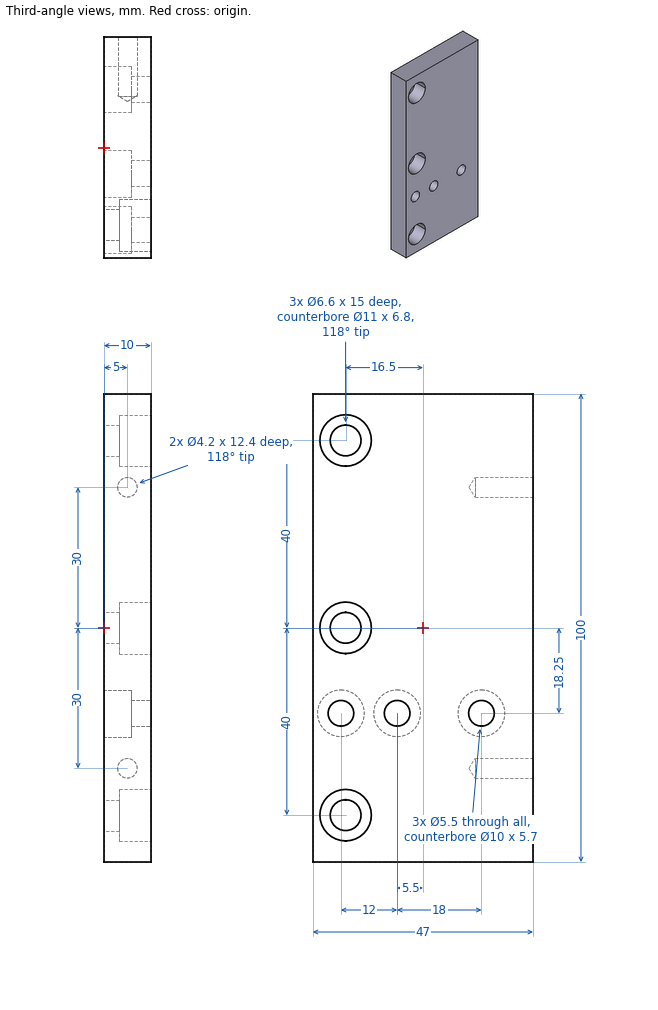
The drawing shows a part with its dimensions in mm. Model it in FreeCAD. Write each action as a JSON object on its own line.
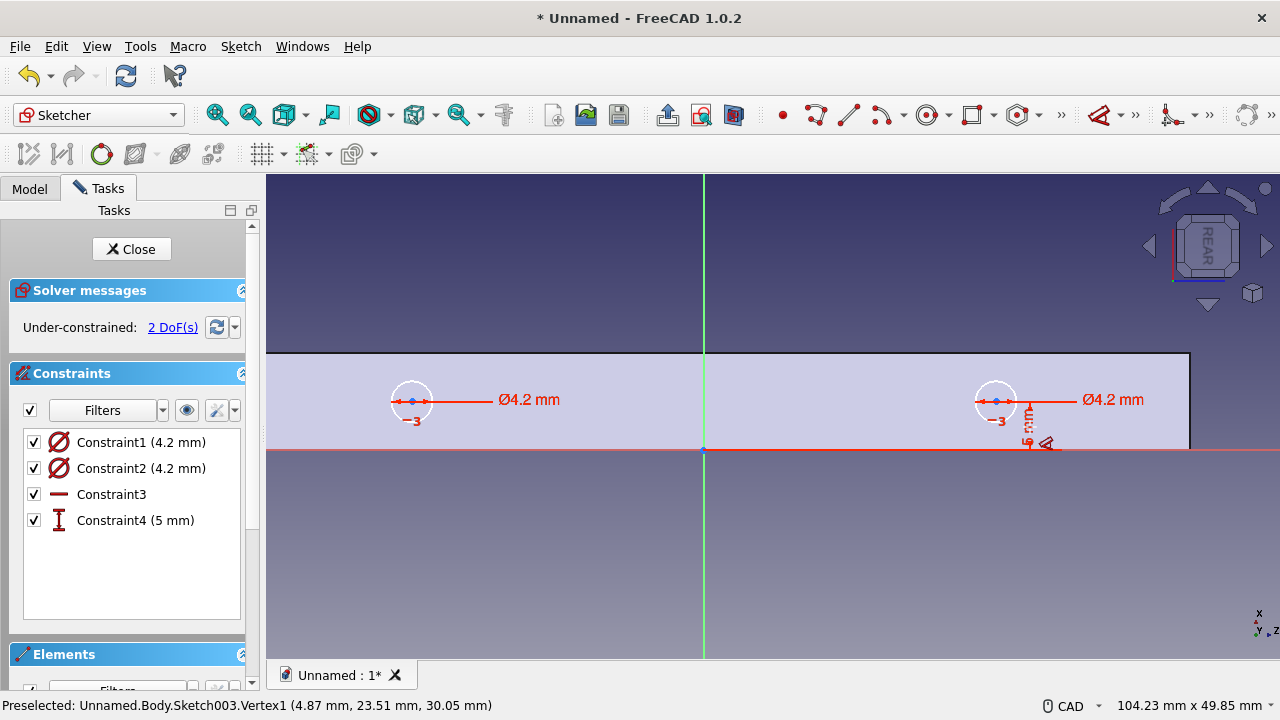
{"action": "left_click", "coordinate": [996, 402]}
{"action": "left_click", "coordinate": [850, 484]}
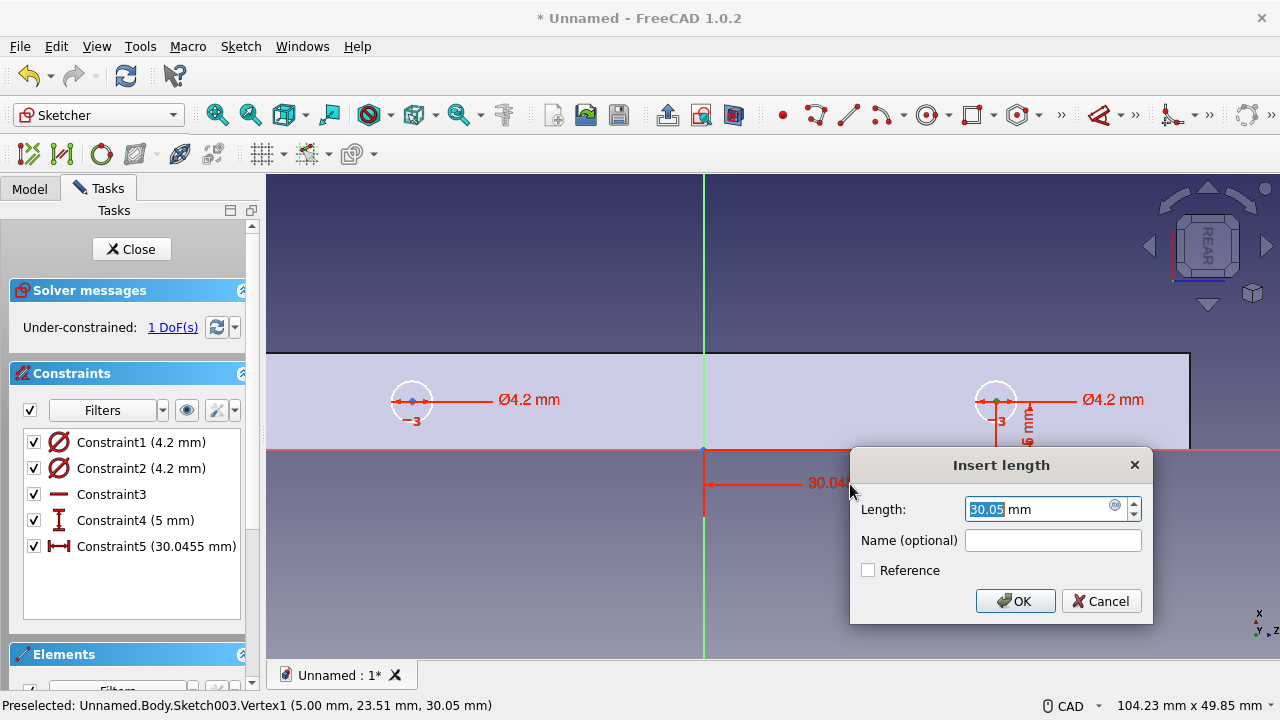
{"action": "type", "text": "30"}
{"action": "key", "text": "Return"}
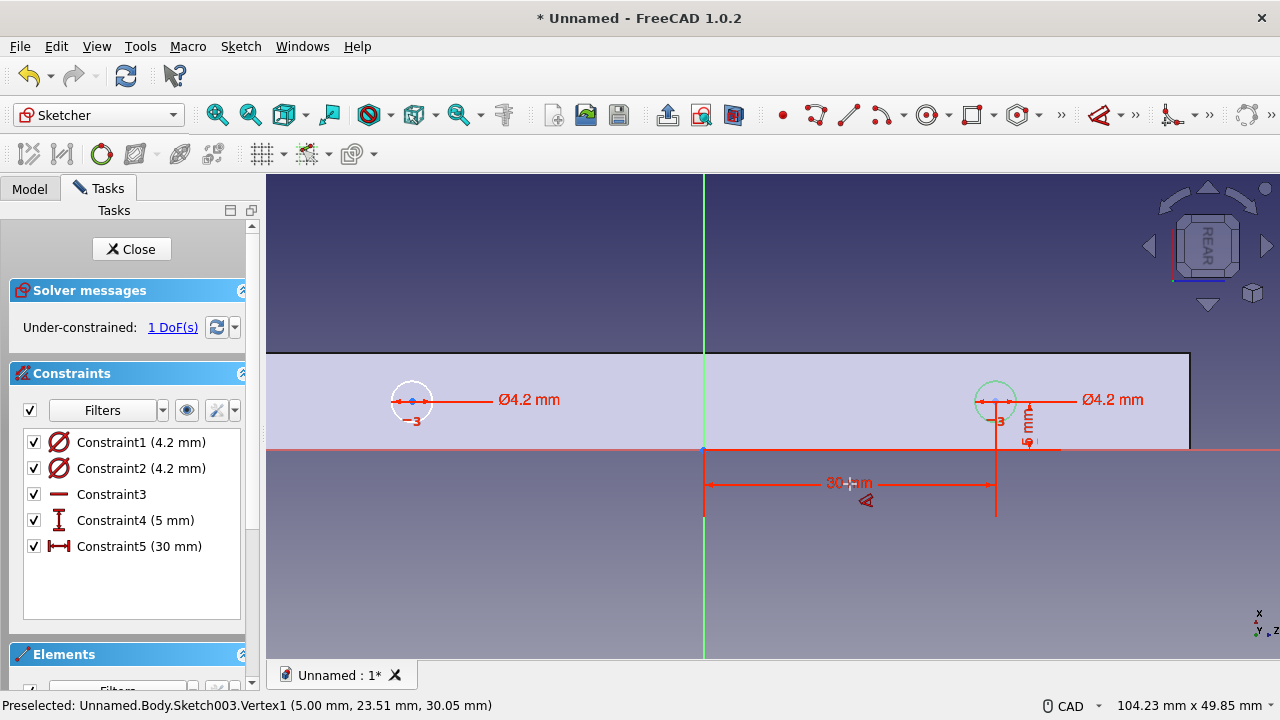
{"action": "left_click", "coordinate": [412, 402]}
{"action": "left_click", "coordinate": [558, 484]}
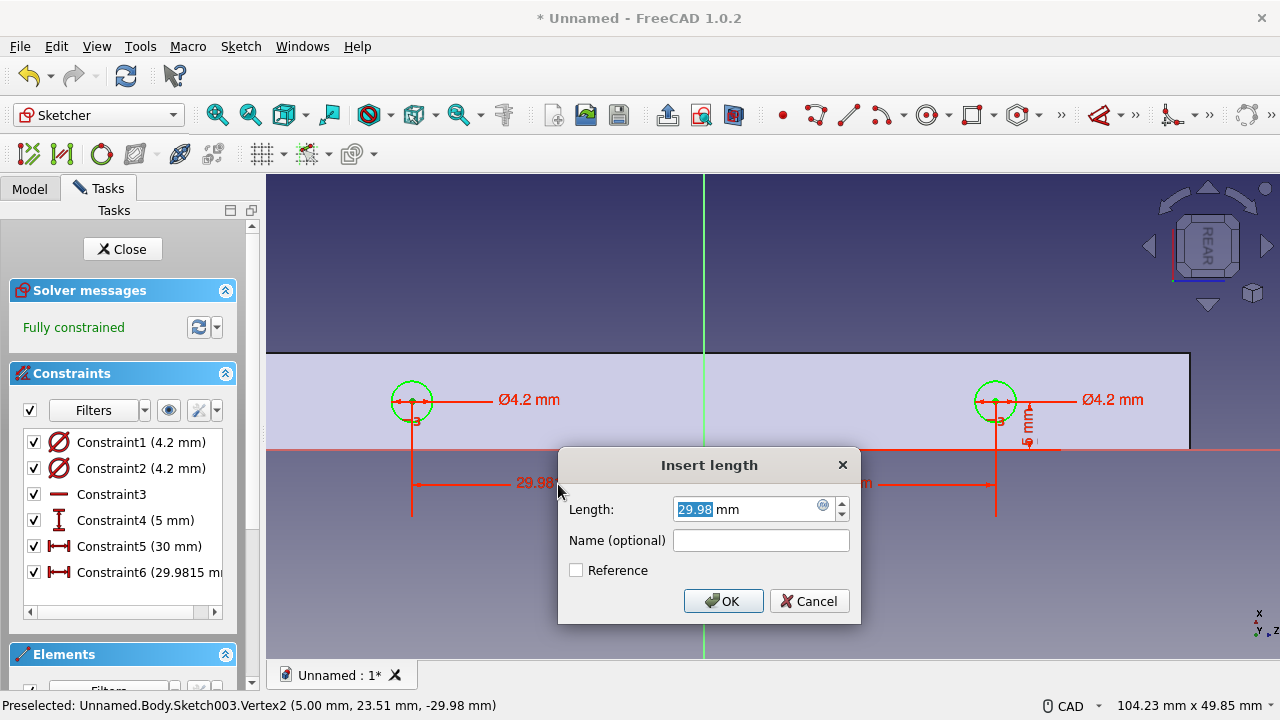
{"action": "type", "text": "30"}
{"action": "key", "text": "Return"}
{"action": "key", "text": "Escape"}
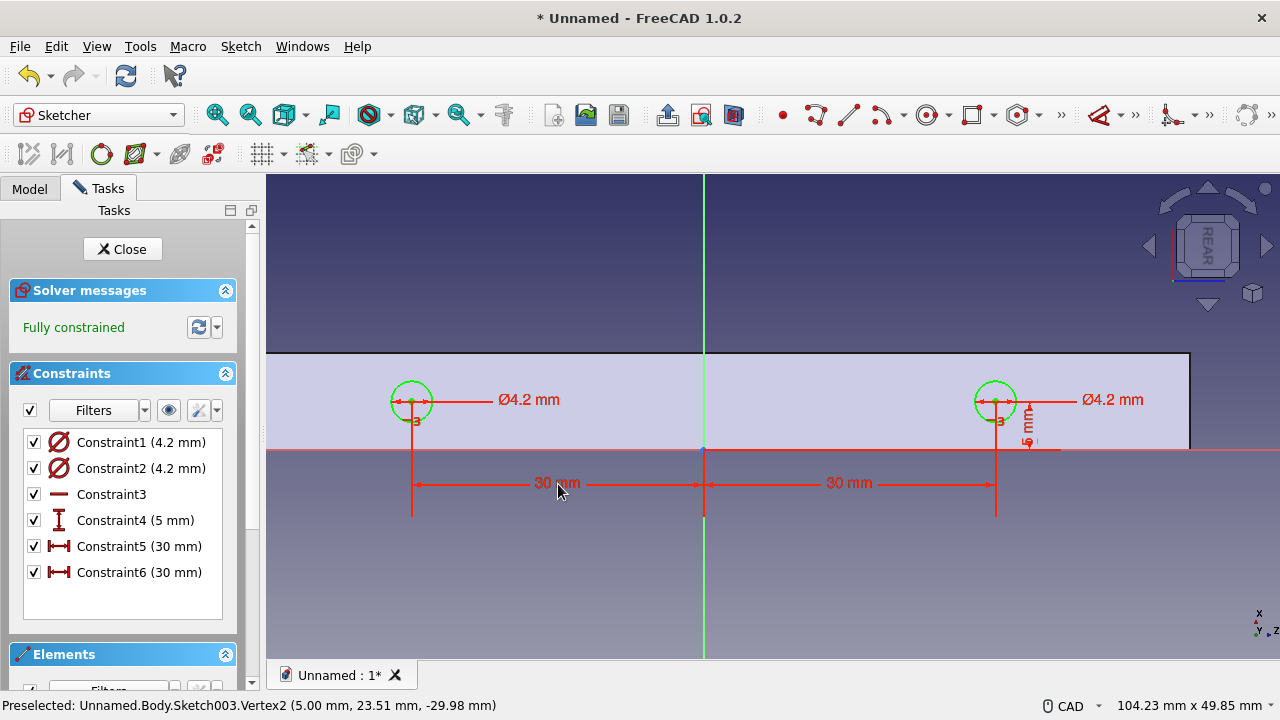
{"action": "left_click", "coordinate": [123, 249]}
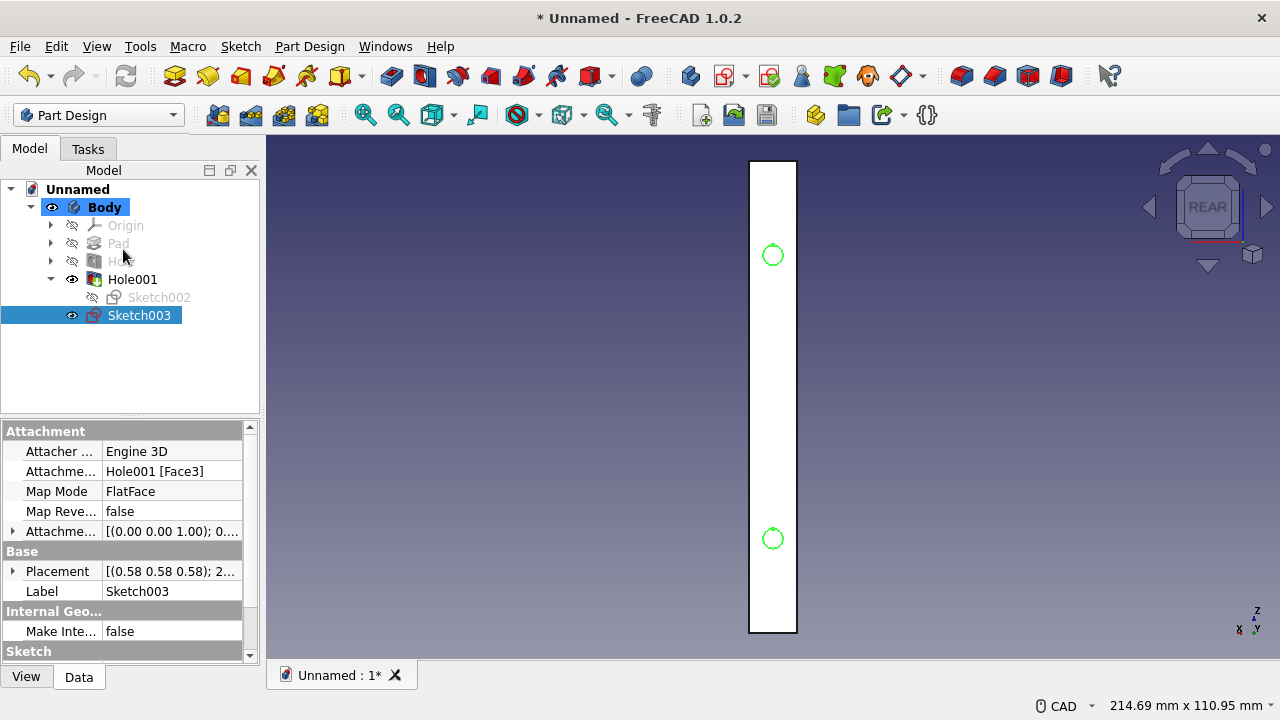
{"action": "left_click", "coordinate": [425, 76]}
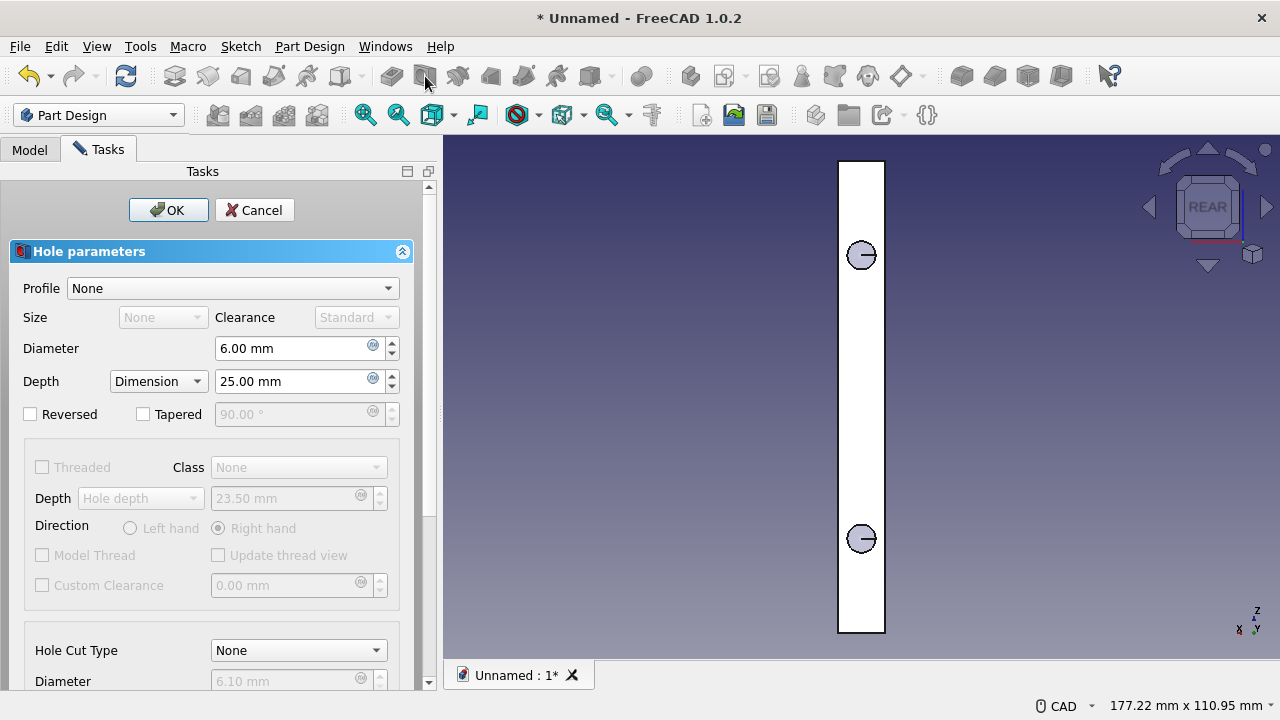
{"action": "triple_click", "coordinate": [300, 348]}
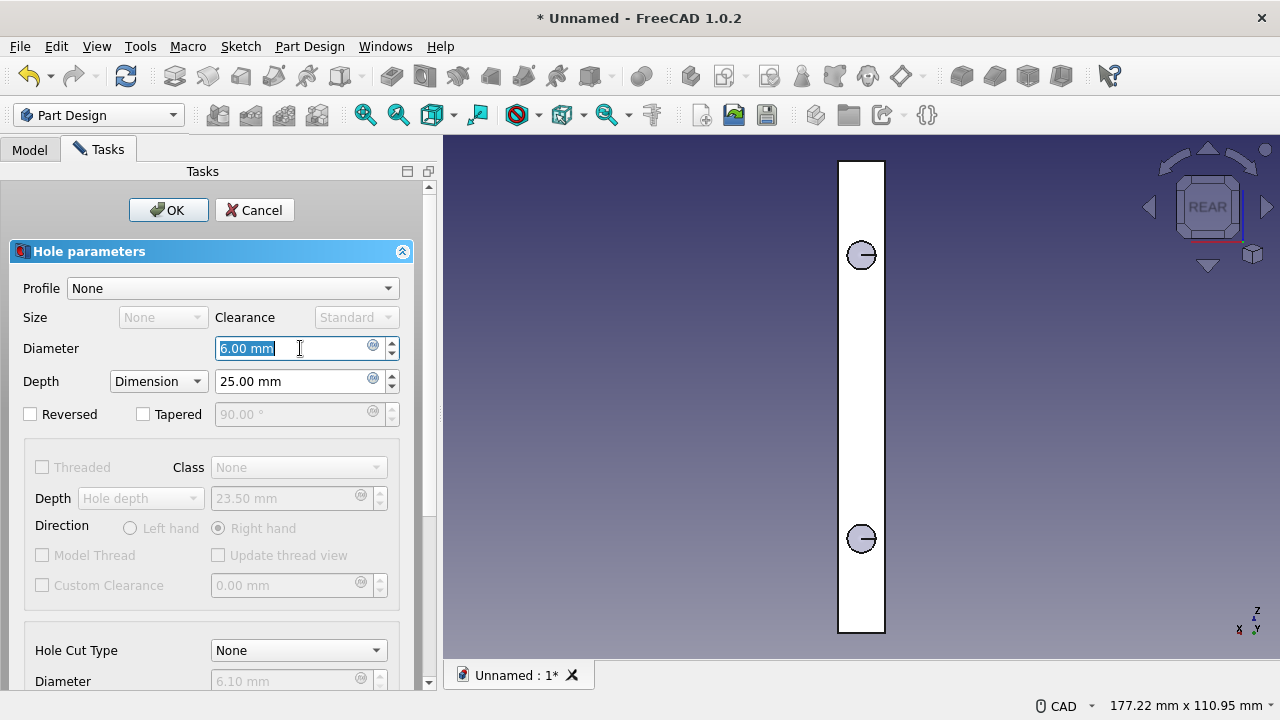
{"action": "type", "text": "4.2"}
{"action": "key", "text": "Tab"}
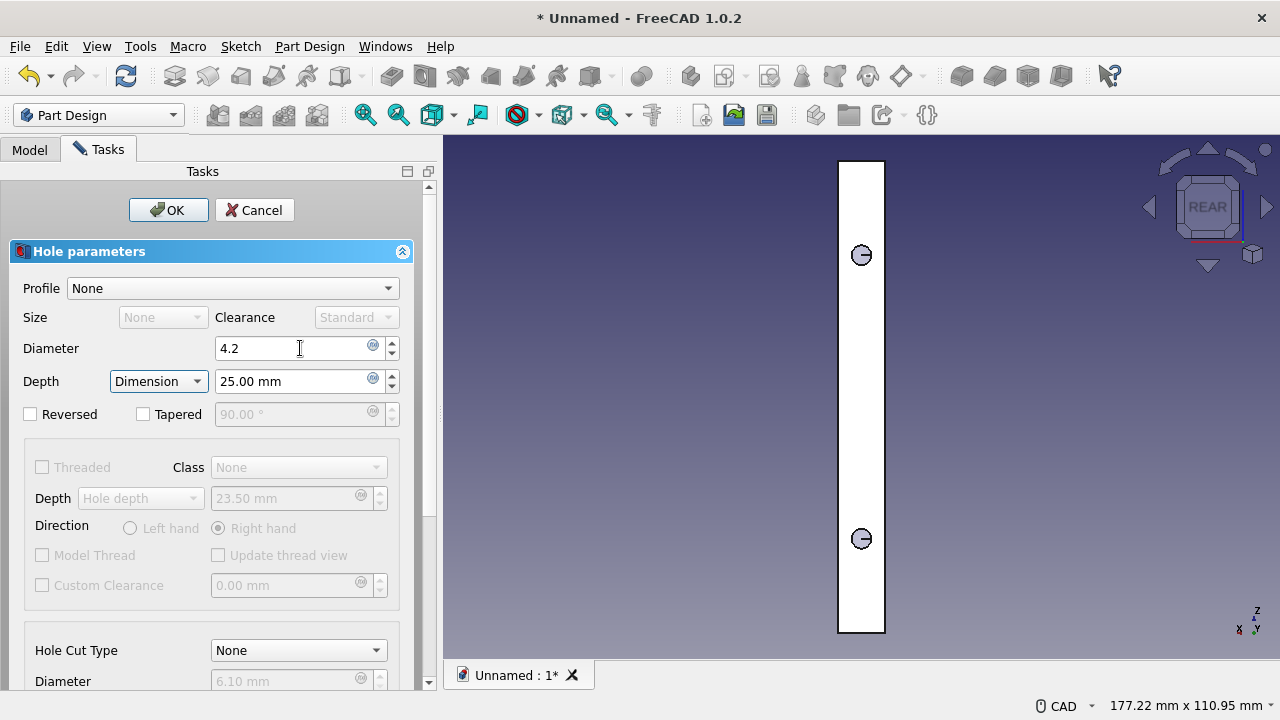
{"action": "triple_click", "coordinate": [300, 382]}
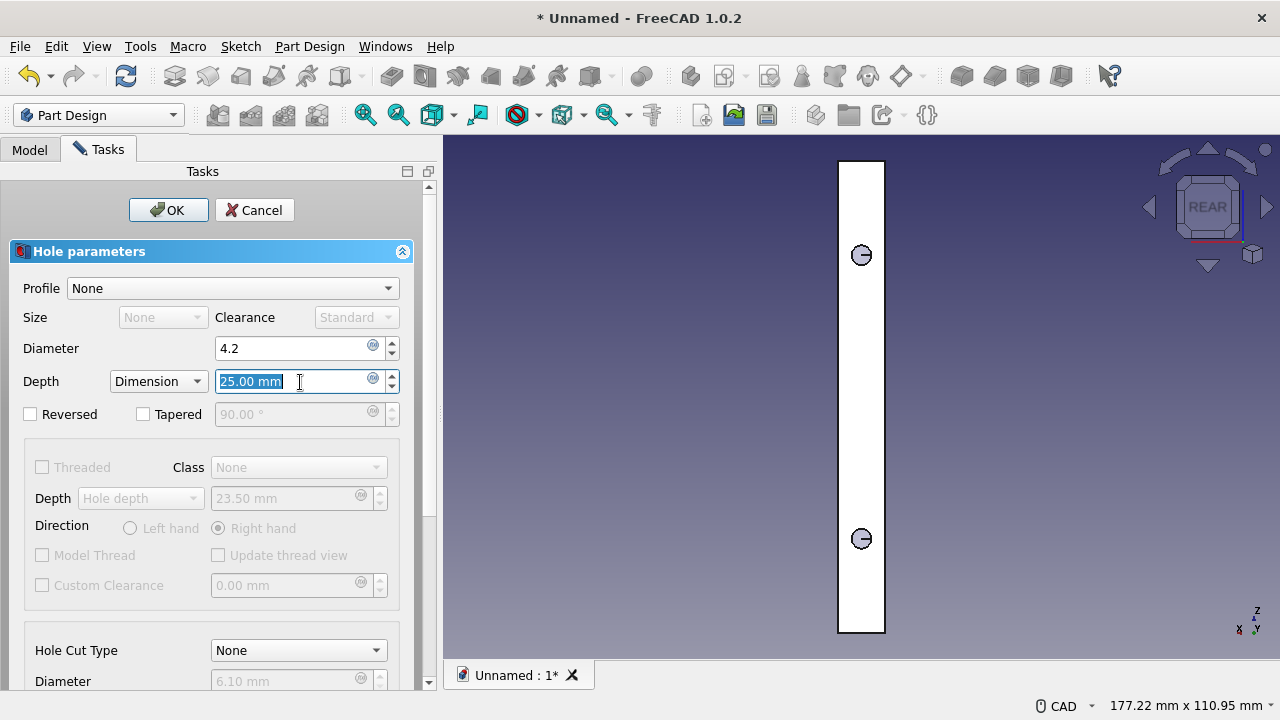
{"action": "type", "text": "12.4"}
{"action": "key", "text": "Tab"}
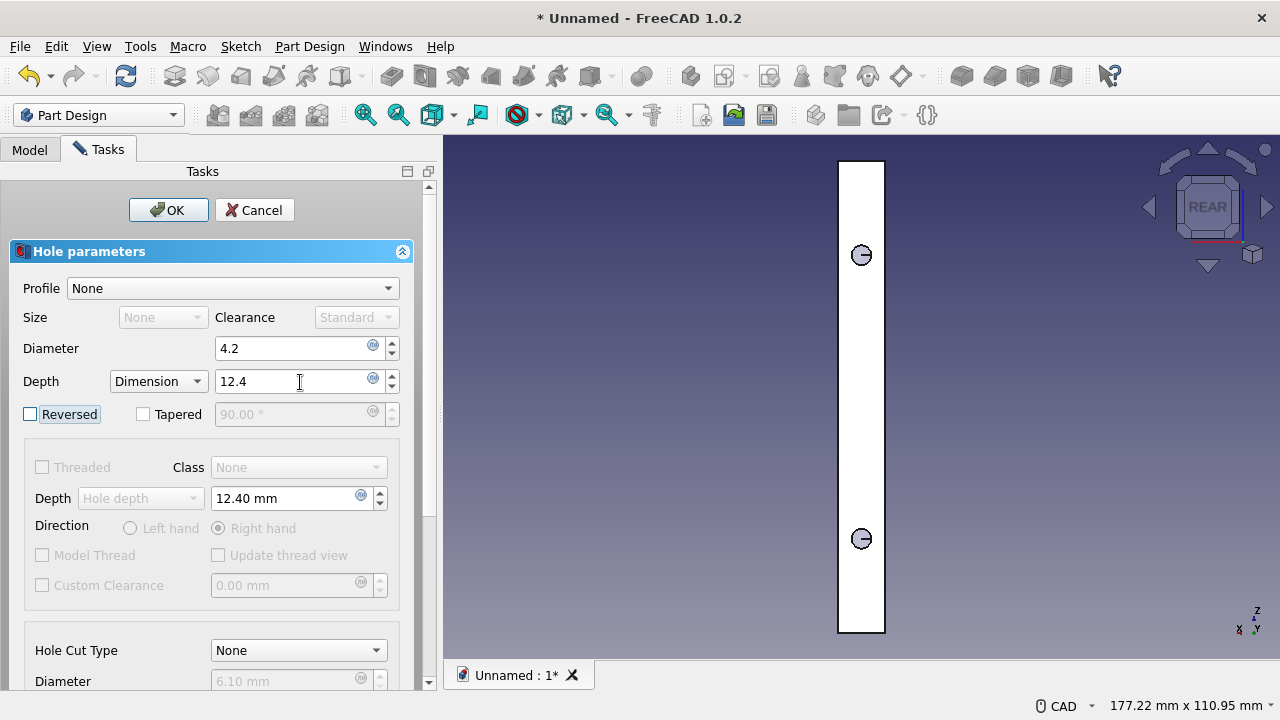
{"action": "left_click", "coordinate": [169, 210]}